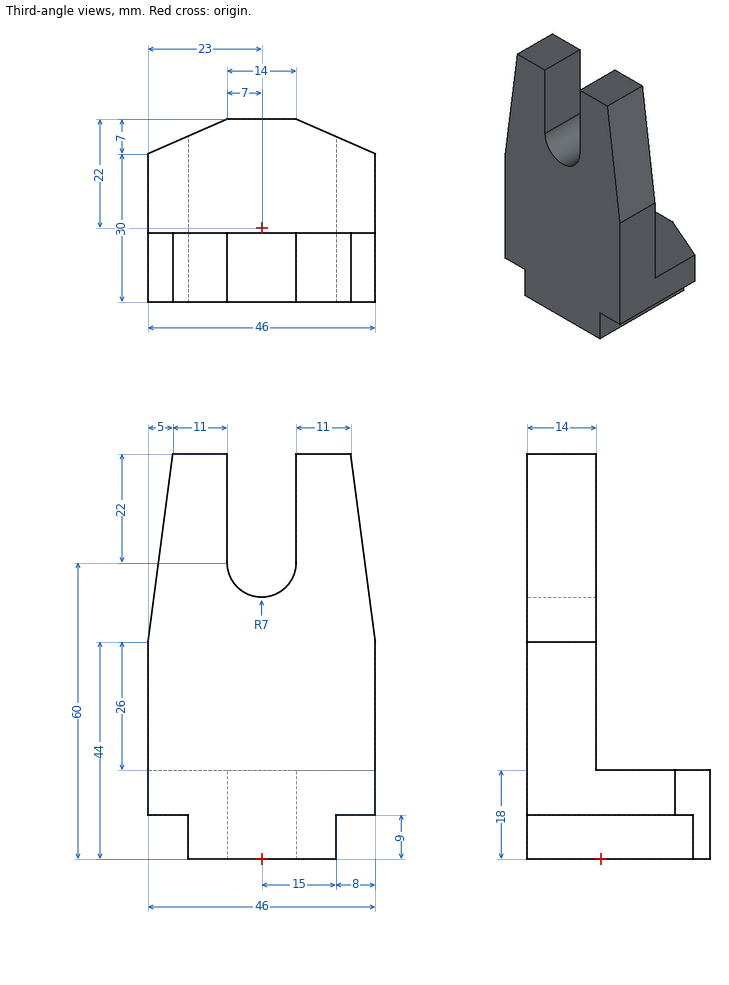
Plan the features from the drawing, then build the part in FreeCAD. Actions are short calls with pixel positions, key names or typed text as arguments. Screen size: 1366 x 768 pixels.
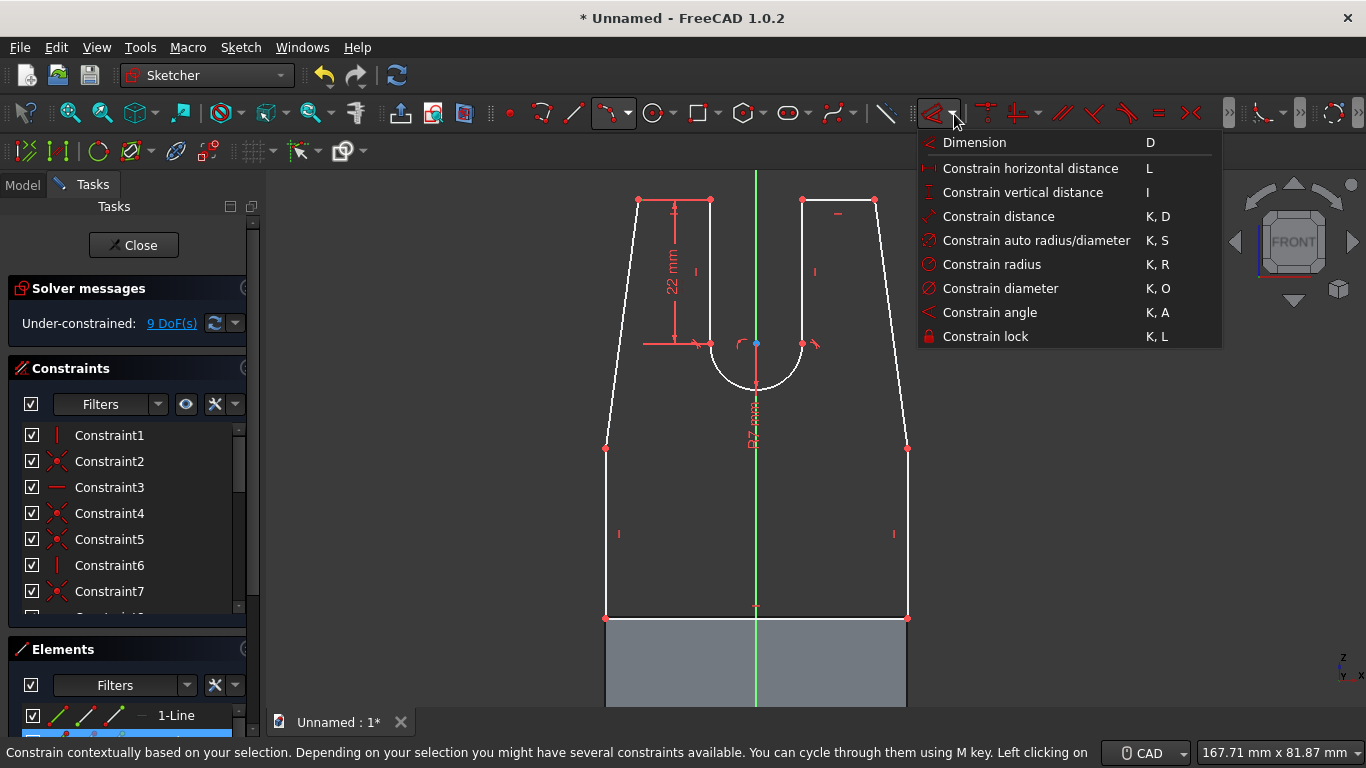
click(1070, 168)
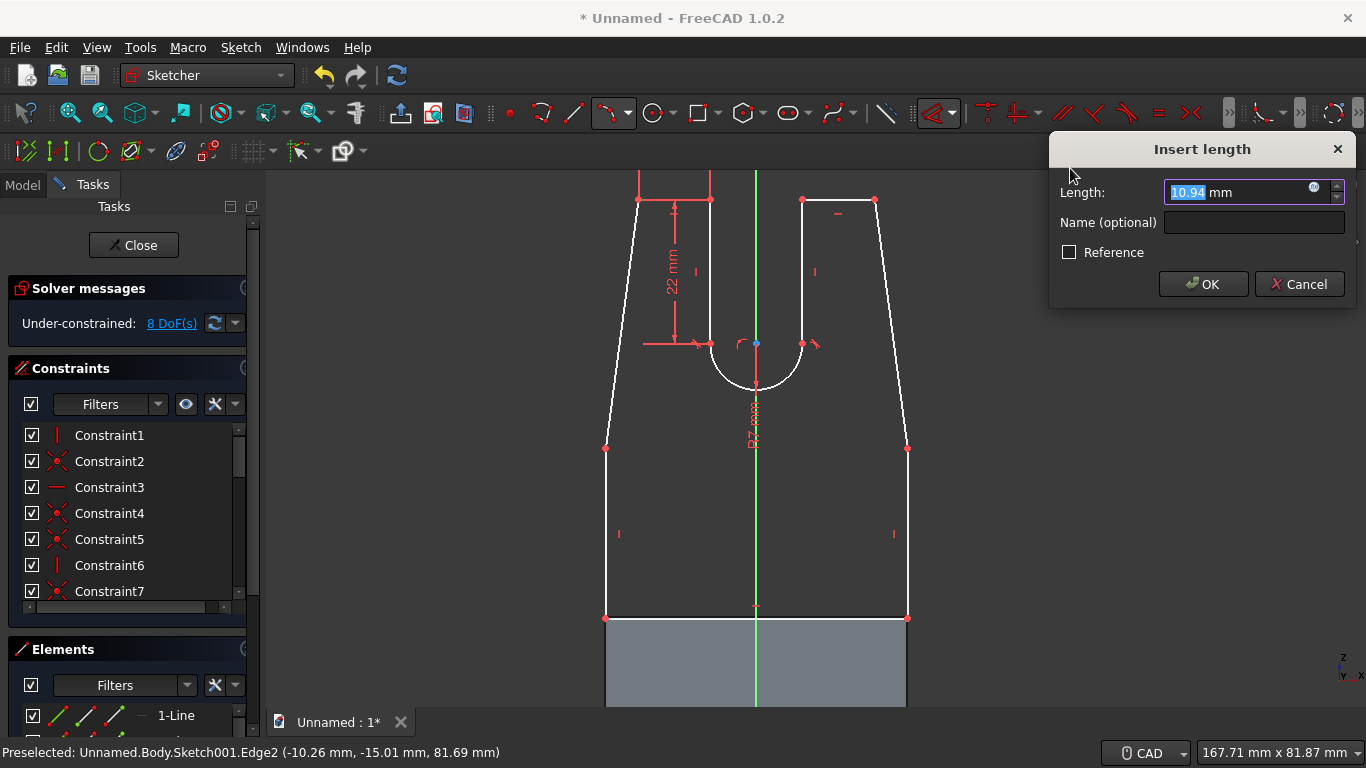
text(11)
key(Return)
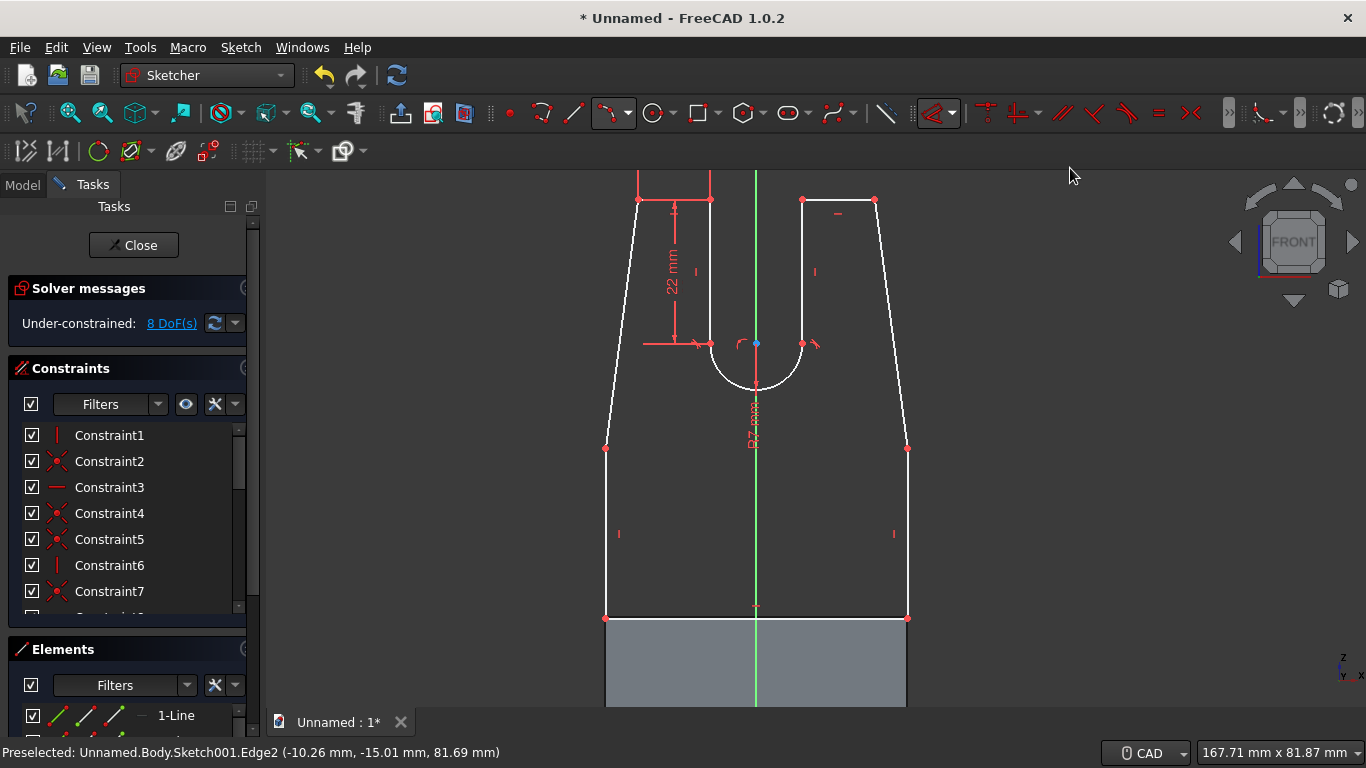
click(606, 499)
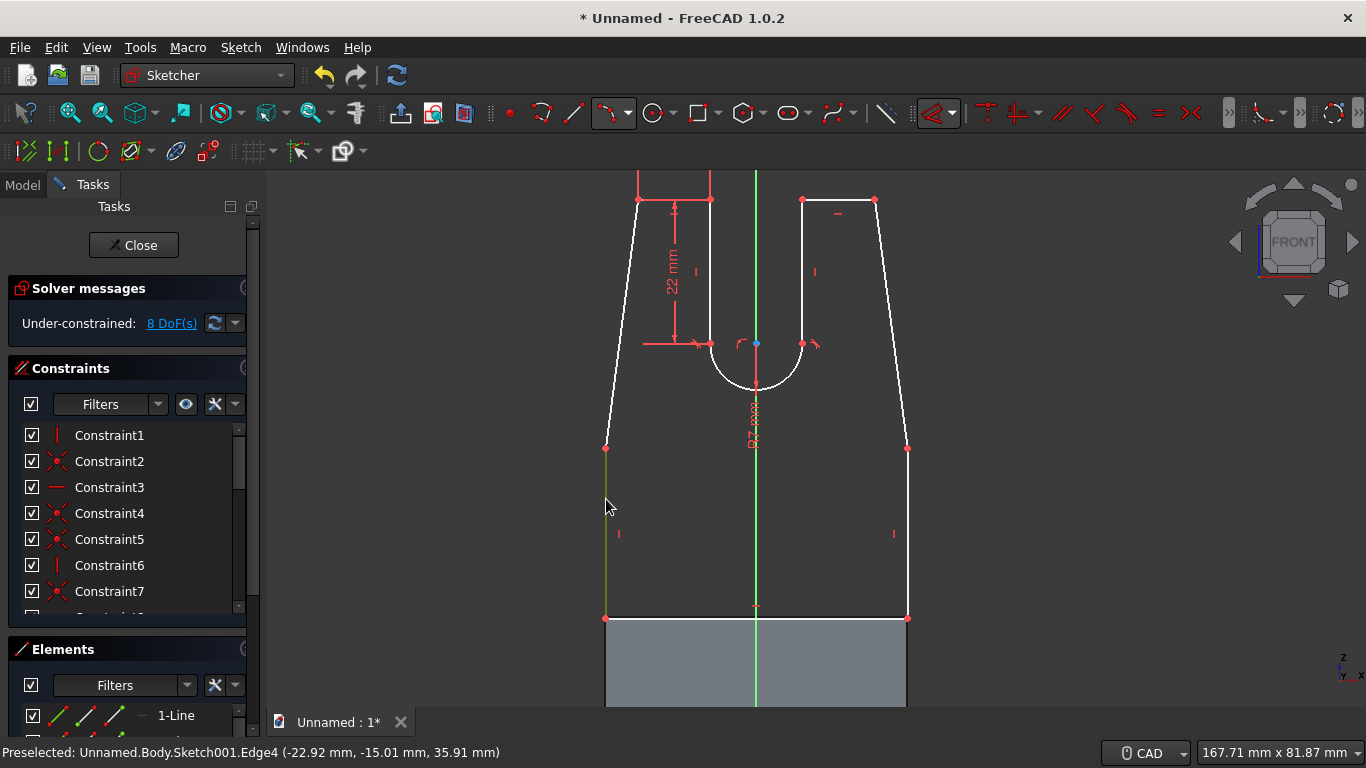
click(954, 114)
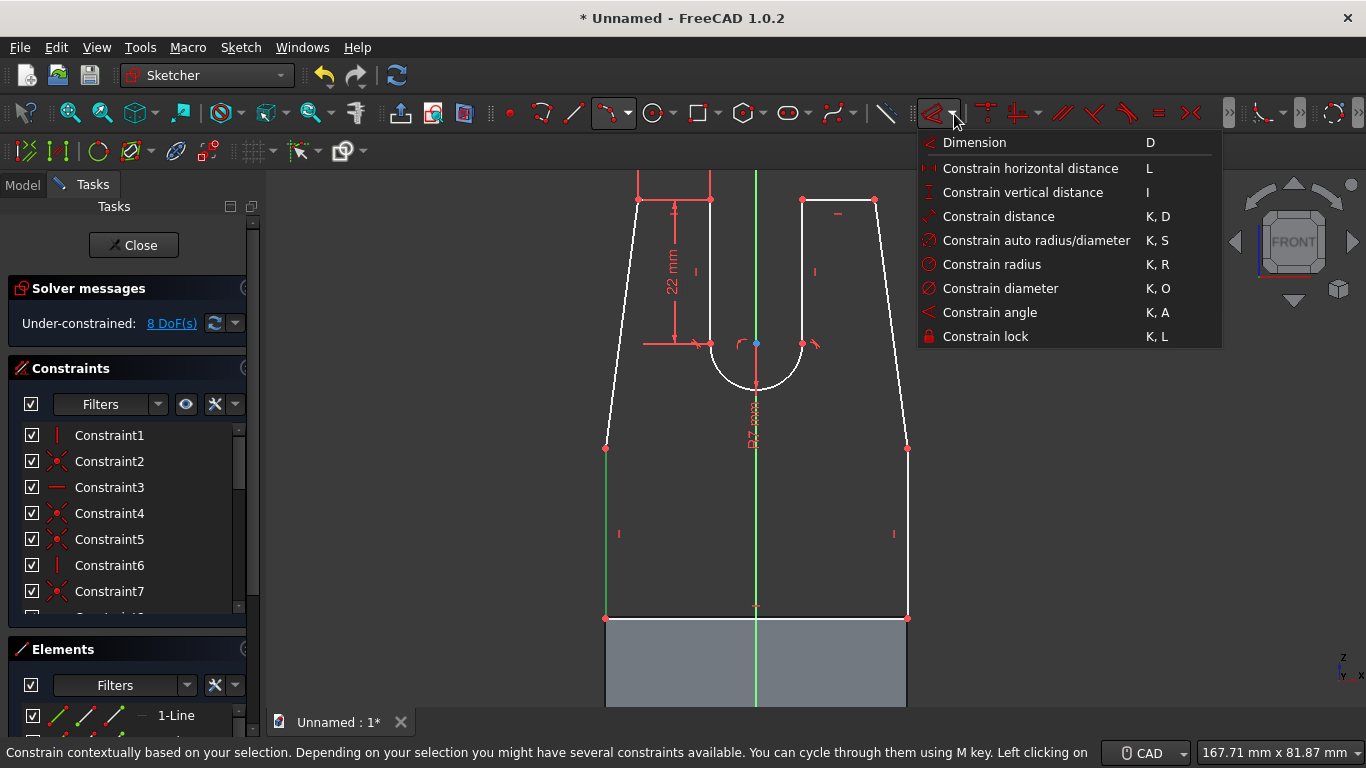
click(1070, 192)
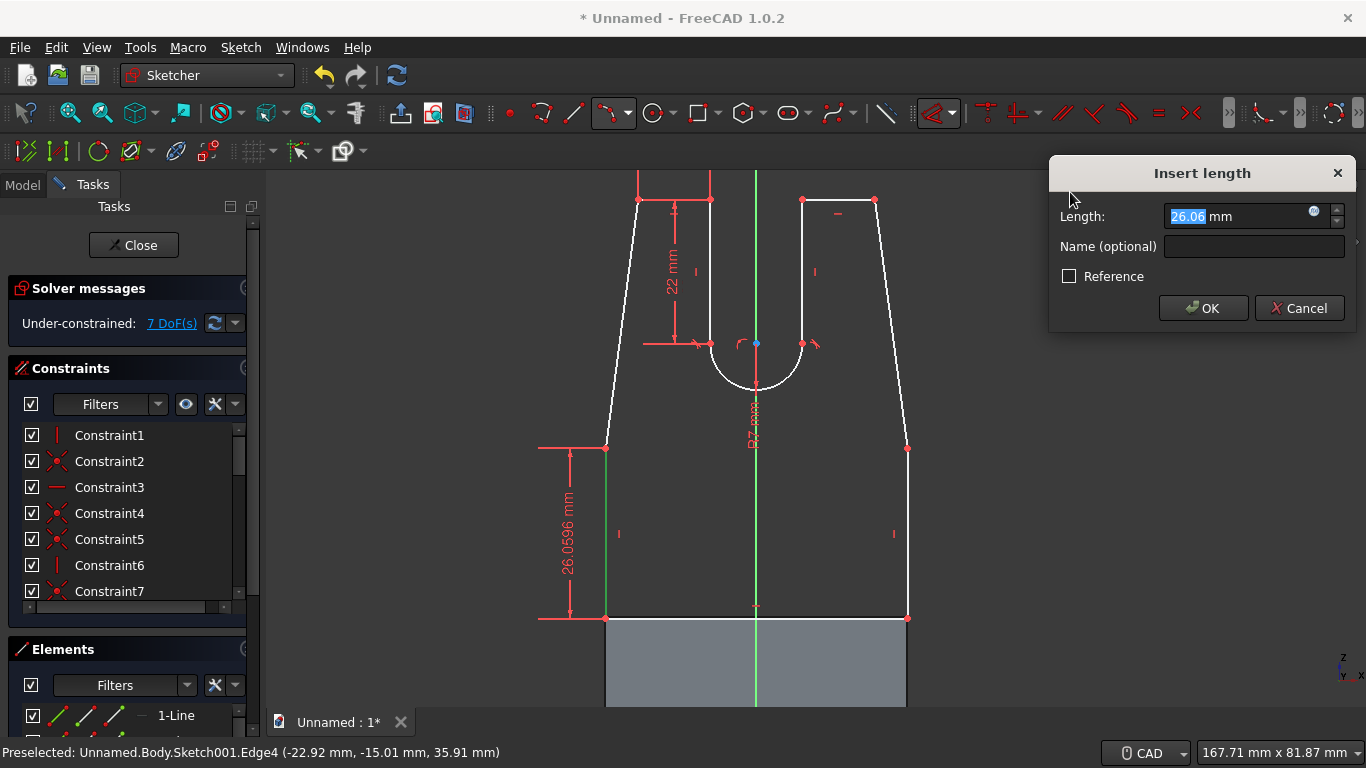
text(26)
key(Return)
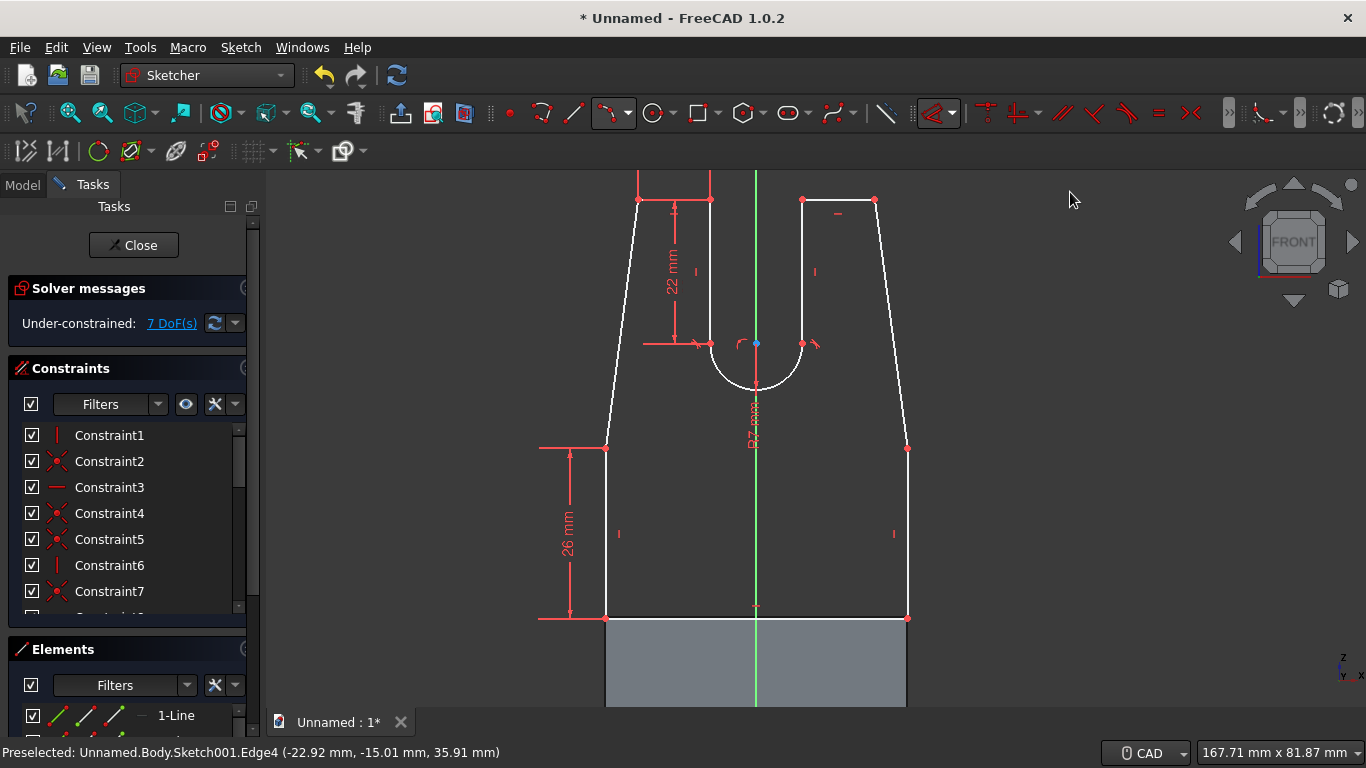
click(696, 619)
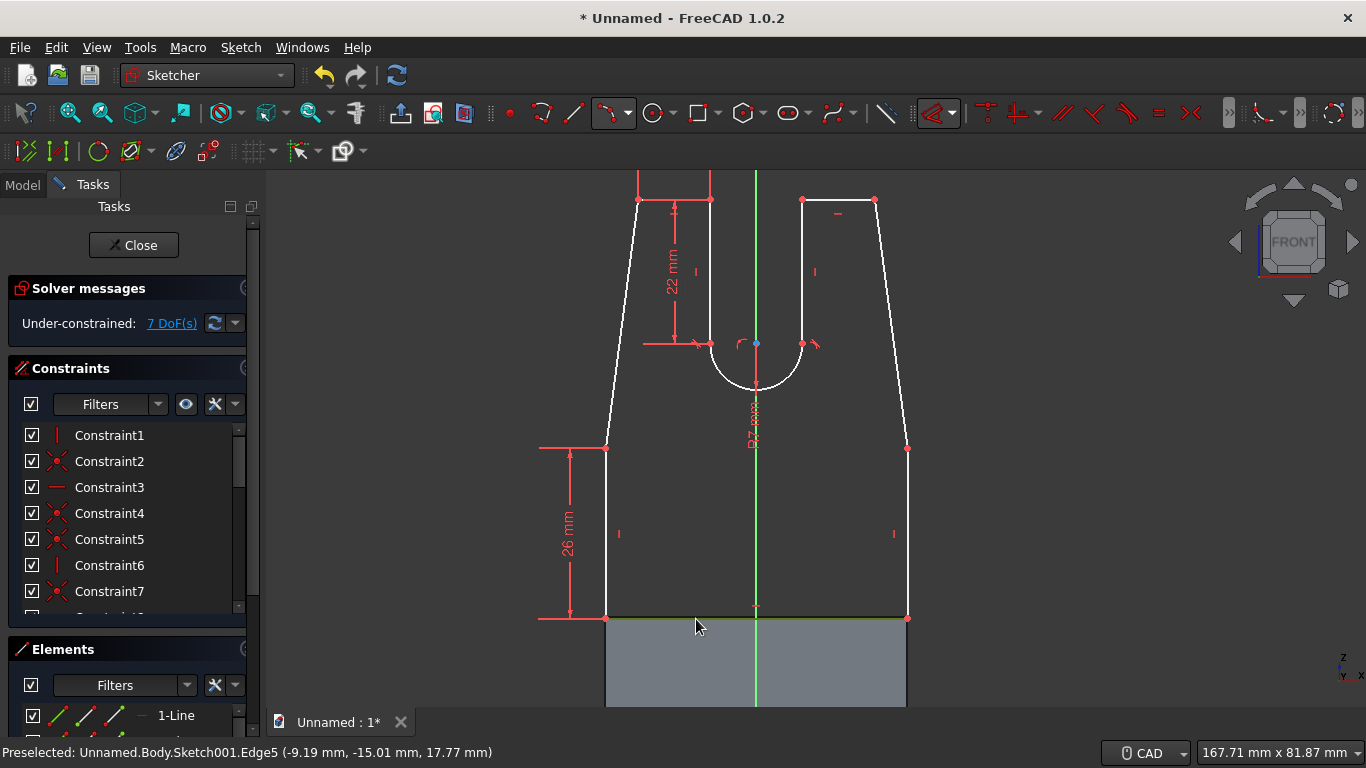
click(954, 114)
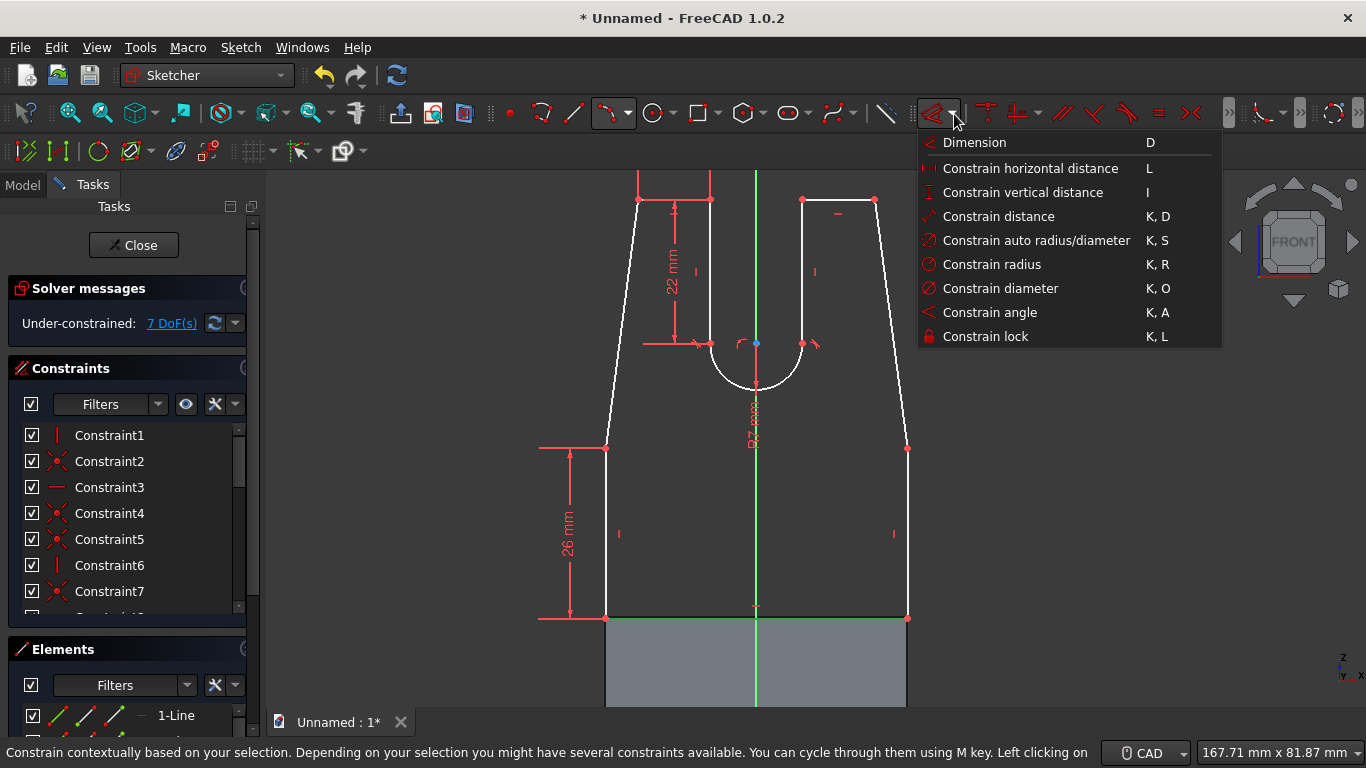
click(1070, 168)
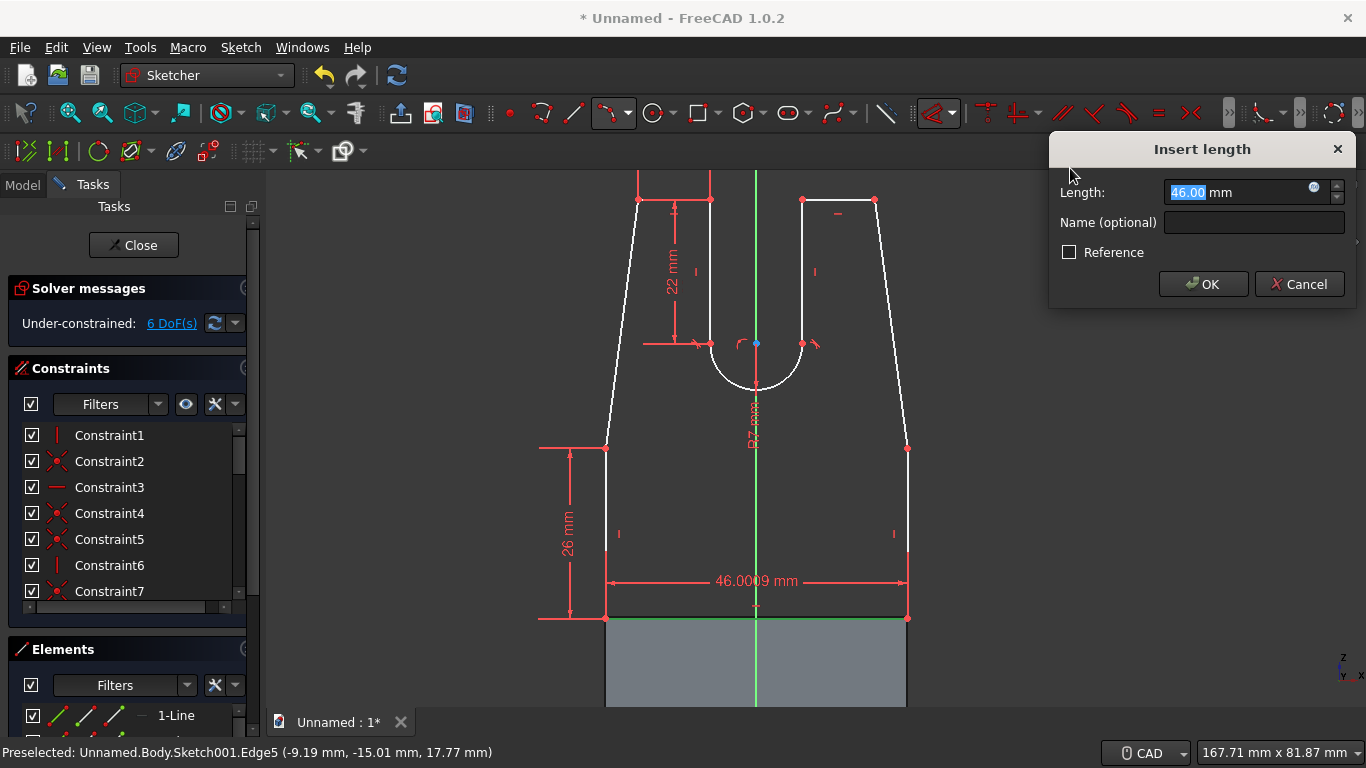
text(46)
key(Return)